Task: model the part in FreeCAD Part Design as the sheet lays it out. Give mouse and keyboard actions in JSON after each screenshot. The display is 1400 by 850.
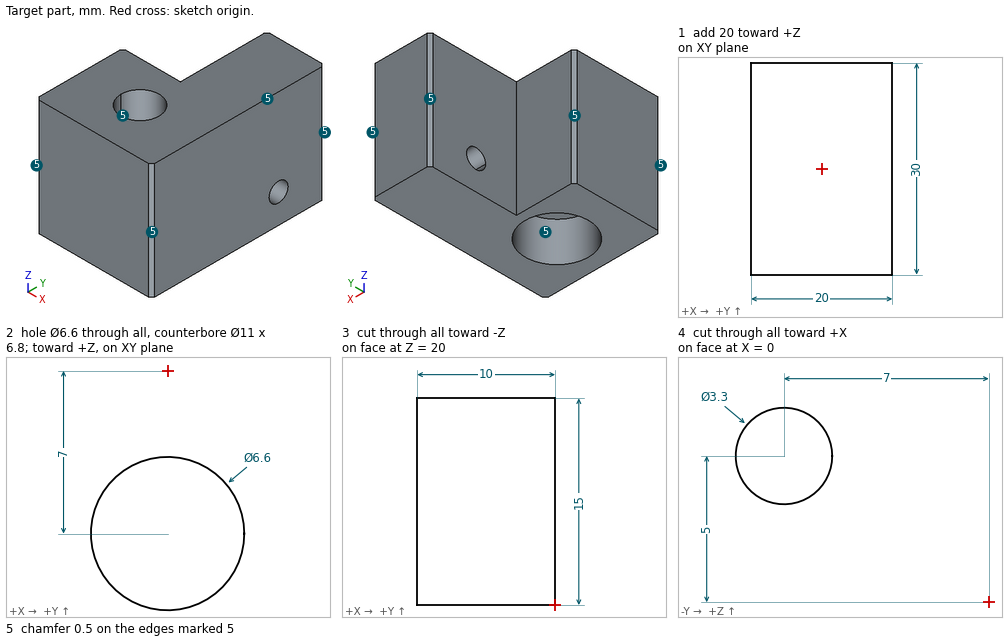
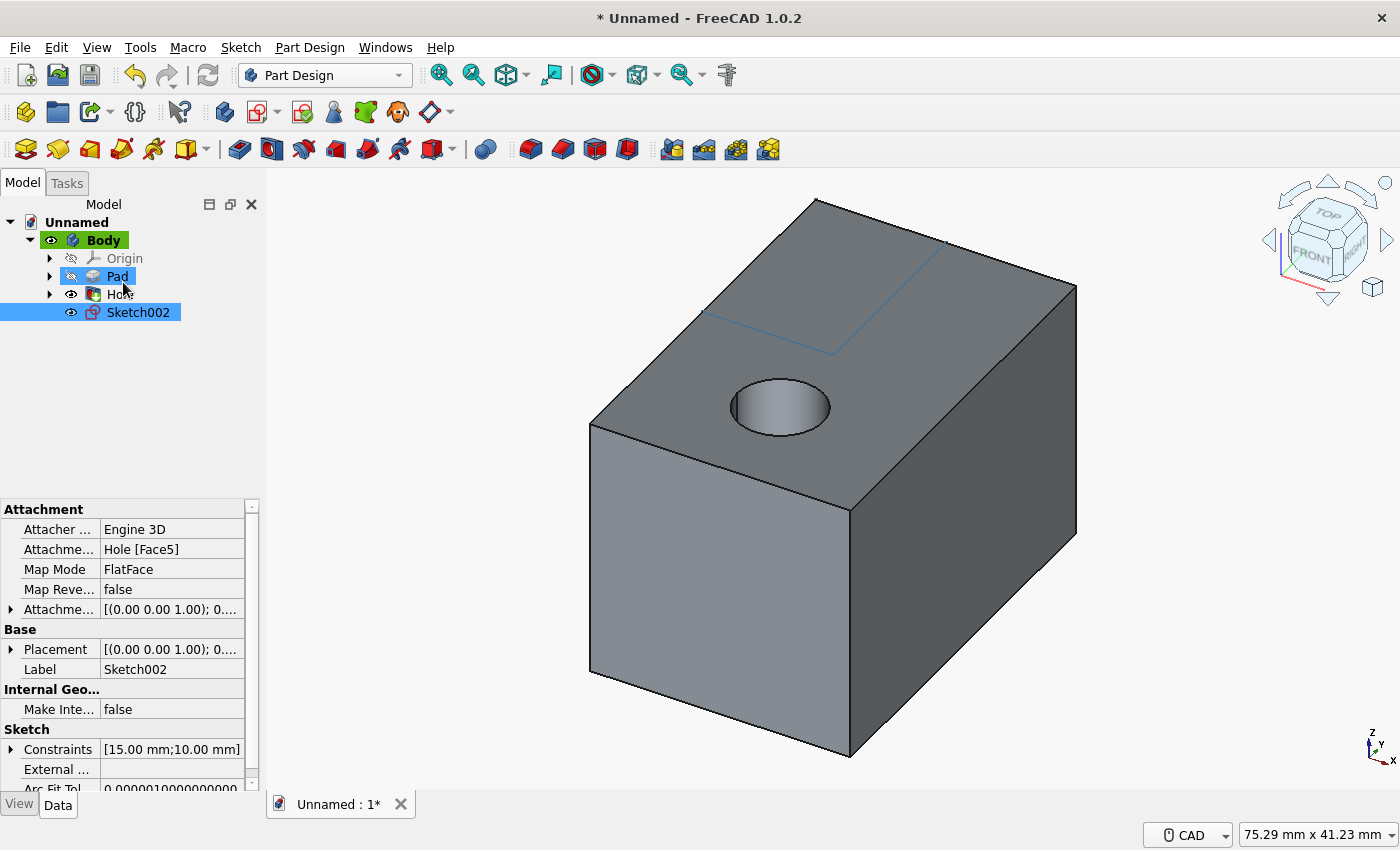
{"action": "left_click", "coordinate": [240, 150]}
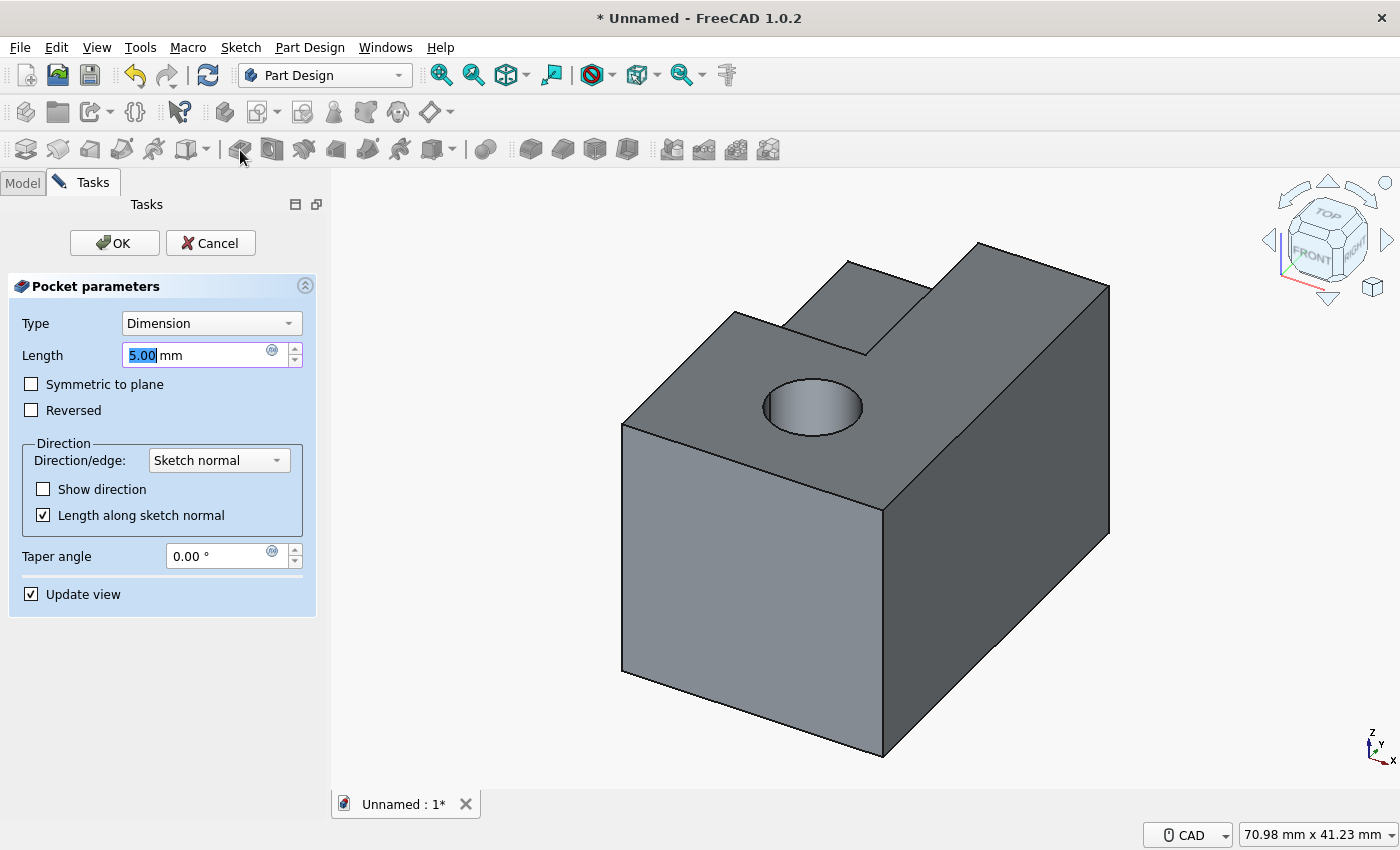
{"action": "left_click", "coordinate": [212, 324]}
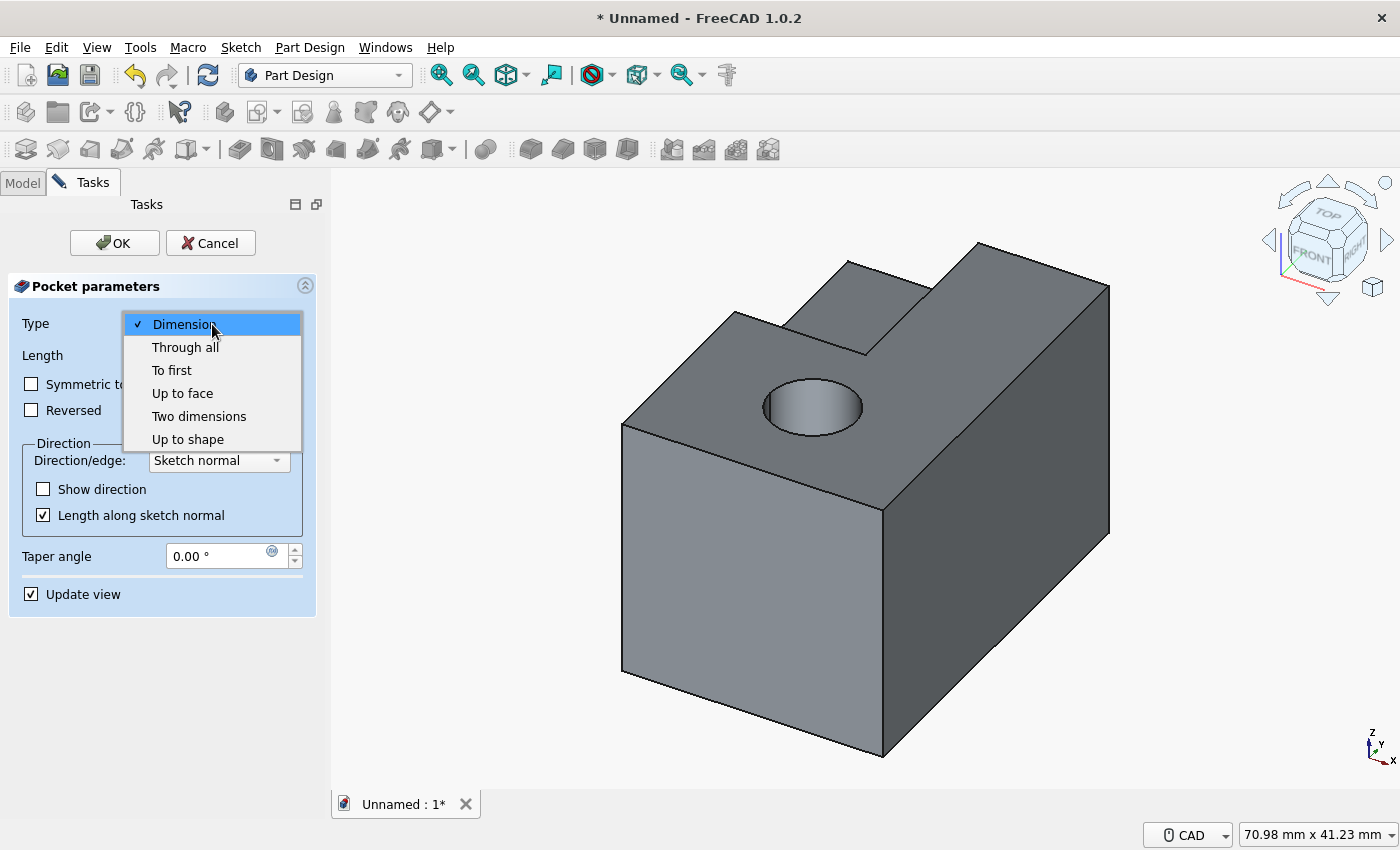
{"action": "left_click", "coordinate": [212, 348]}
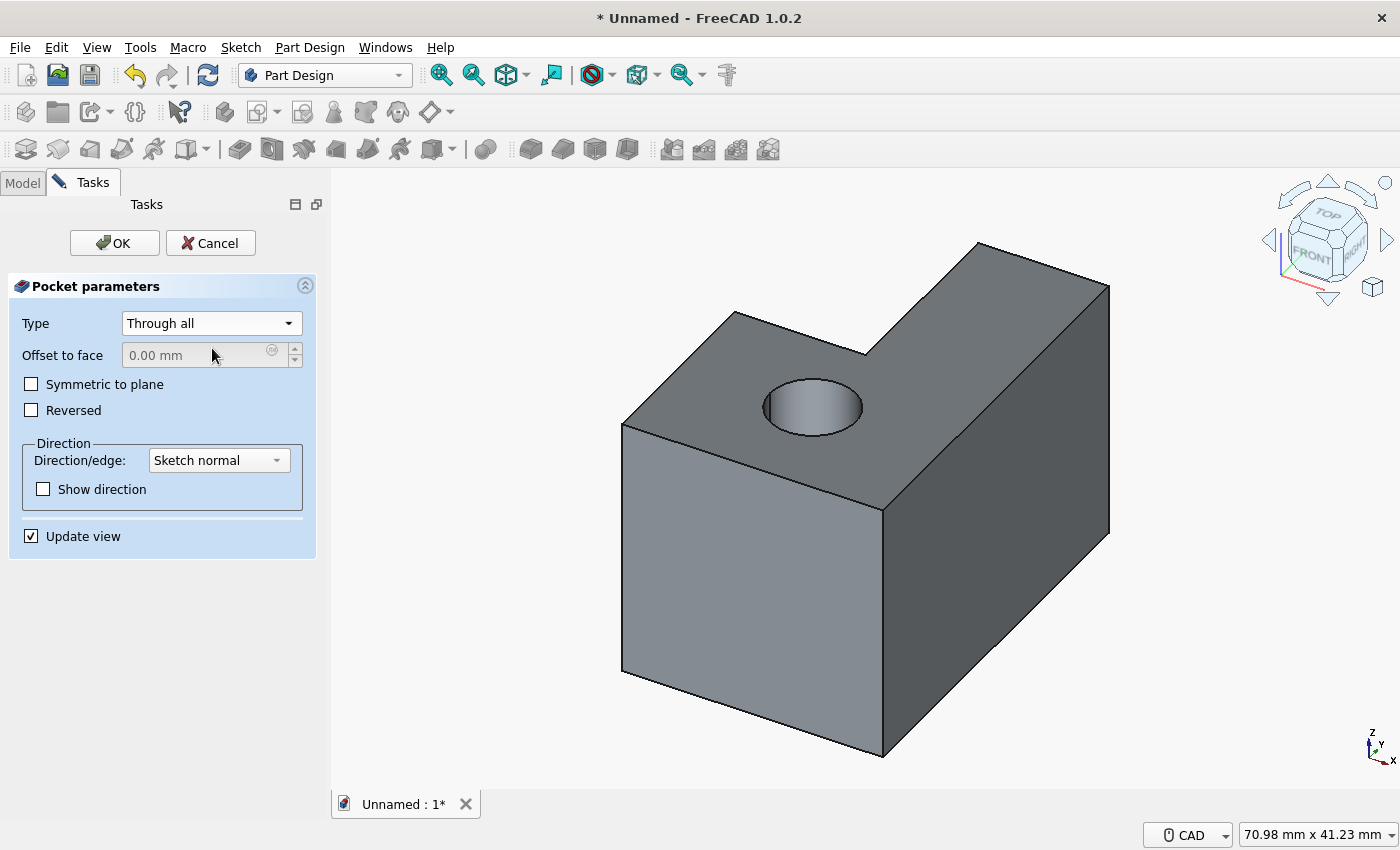
{"action": "left_click", "coordinate": [115, 243]}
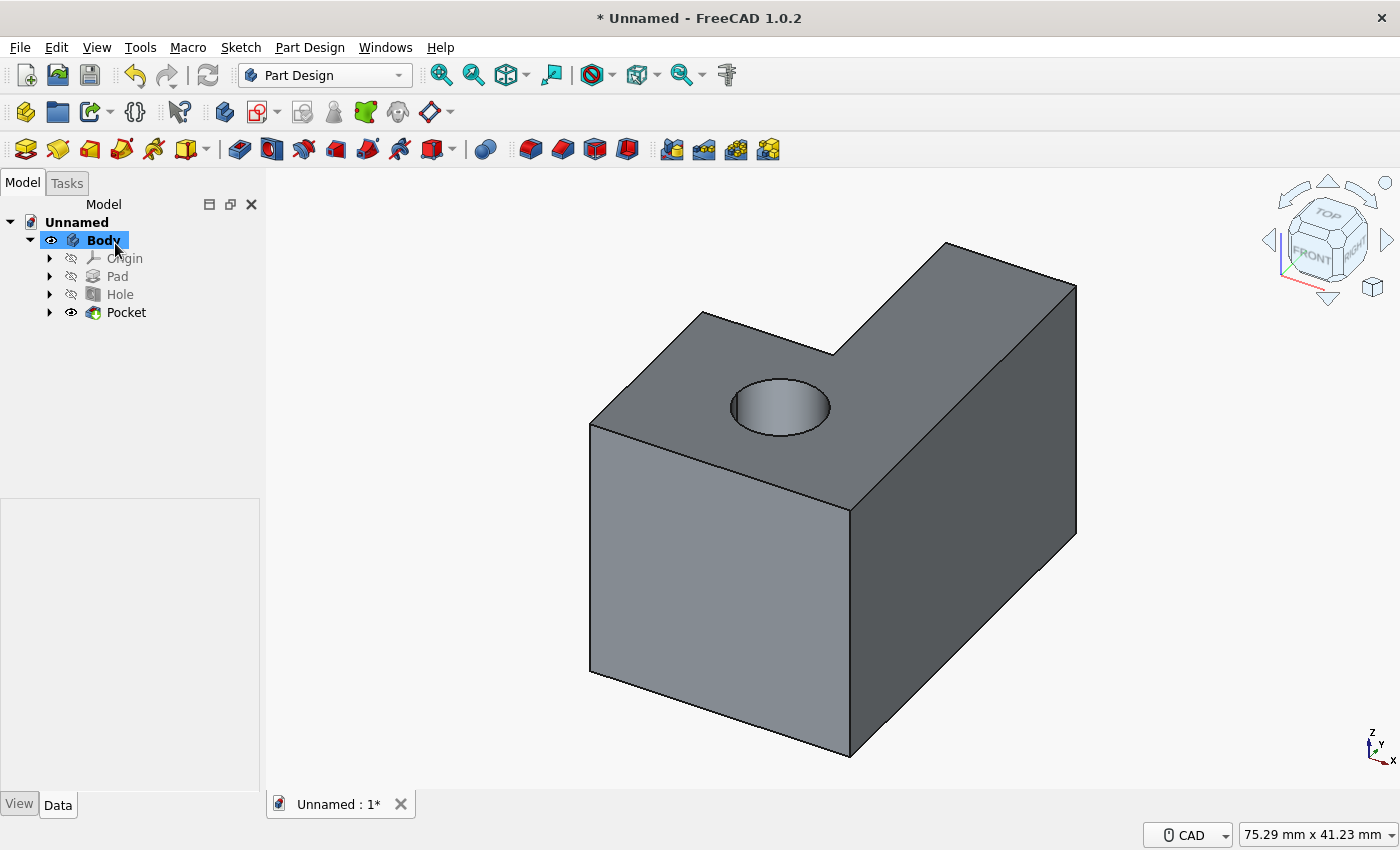
{"action": "key", "text": "6"}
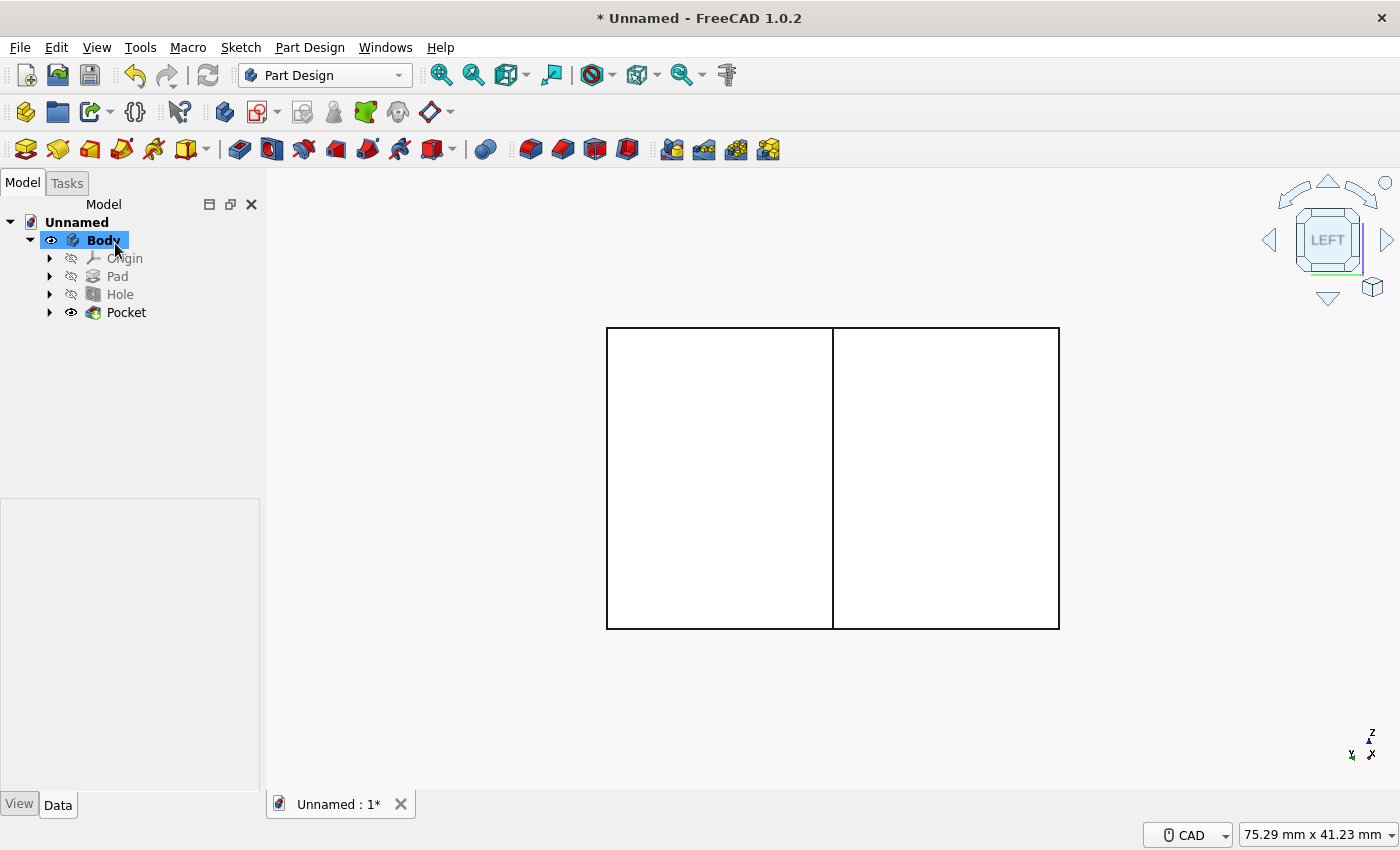
{"action": "left_click", "coordinate": [720, 477]}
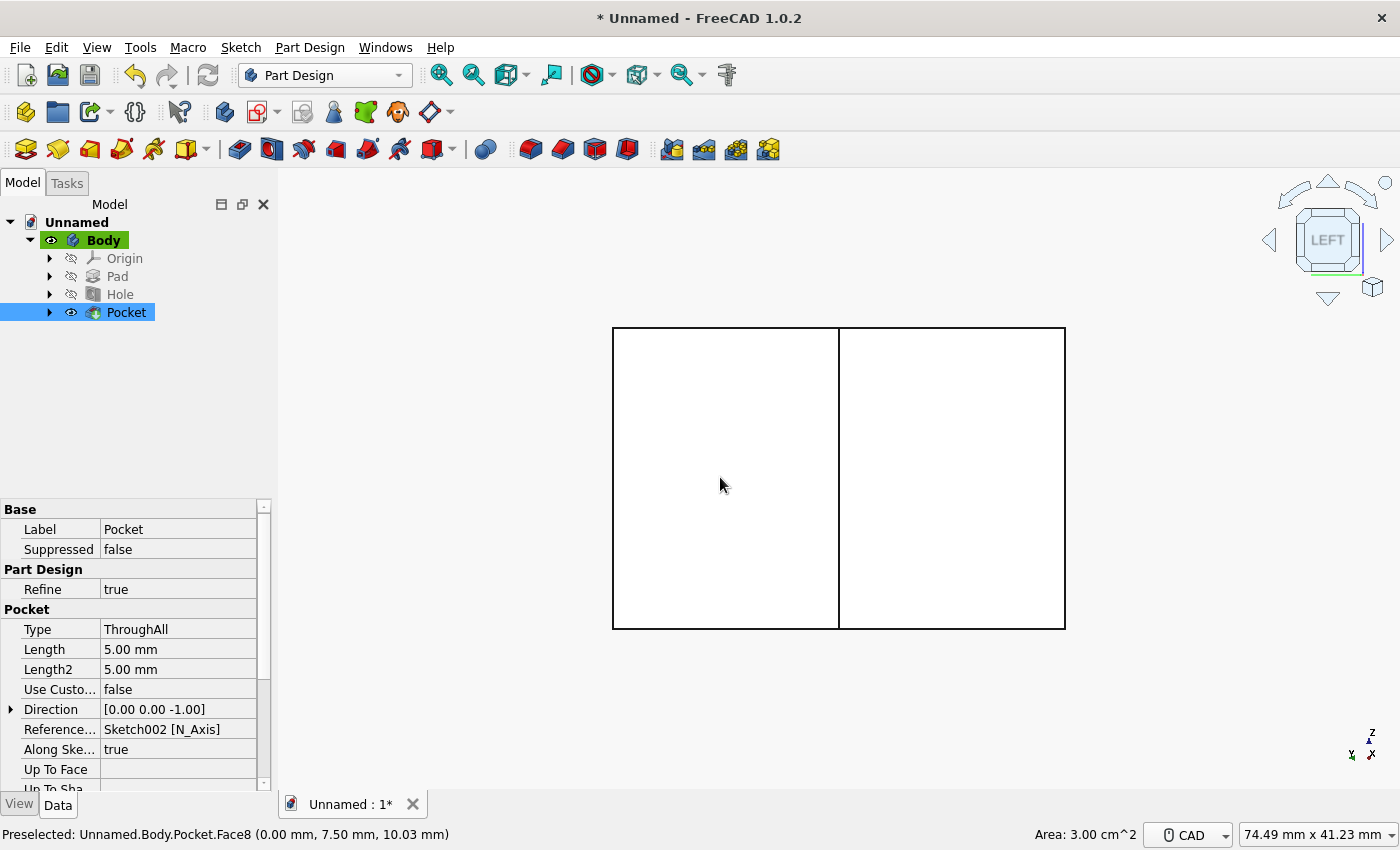
{"action": "left_click", "coordinate": [258, 112]}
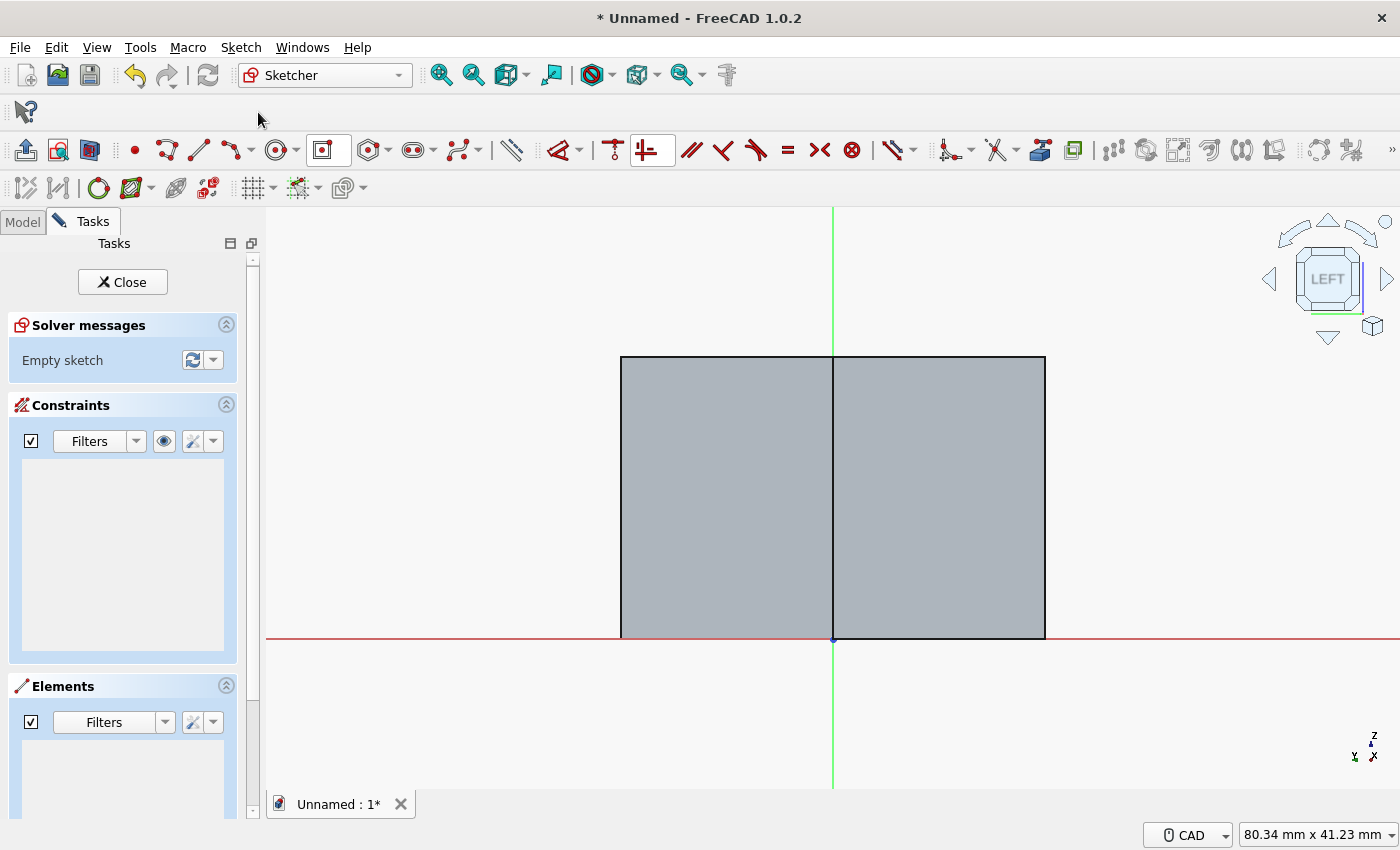
{"action": "scroll", "coordinate": [729, 580], "scroll_direction": "up", "scroll_amount": 10}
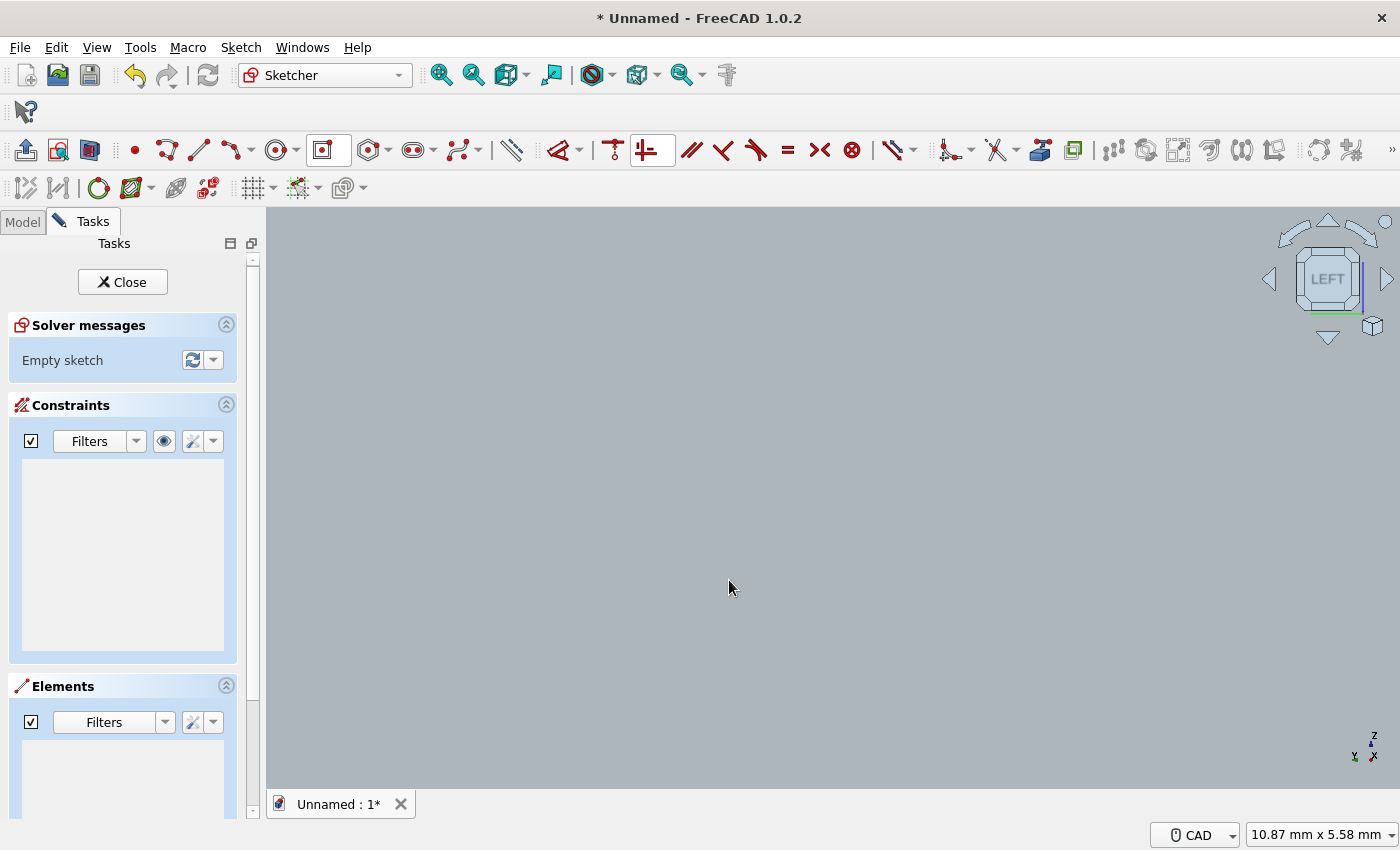
{"action": "left_click", "coordinate": [276, 150]}